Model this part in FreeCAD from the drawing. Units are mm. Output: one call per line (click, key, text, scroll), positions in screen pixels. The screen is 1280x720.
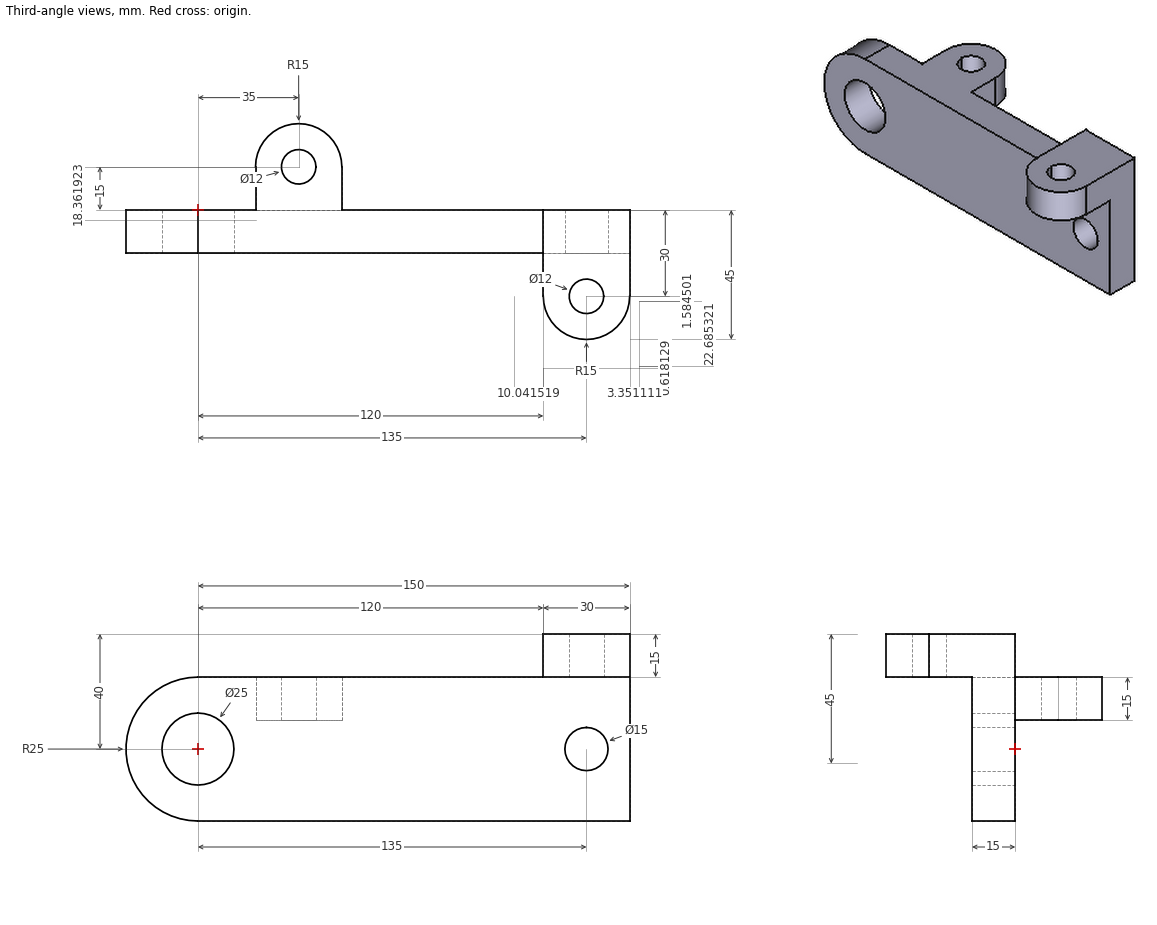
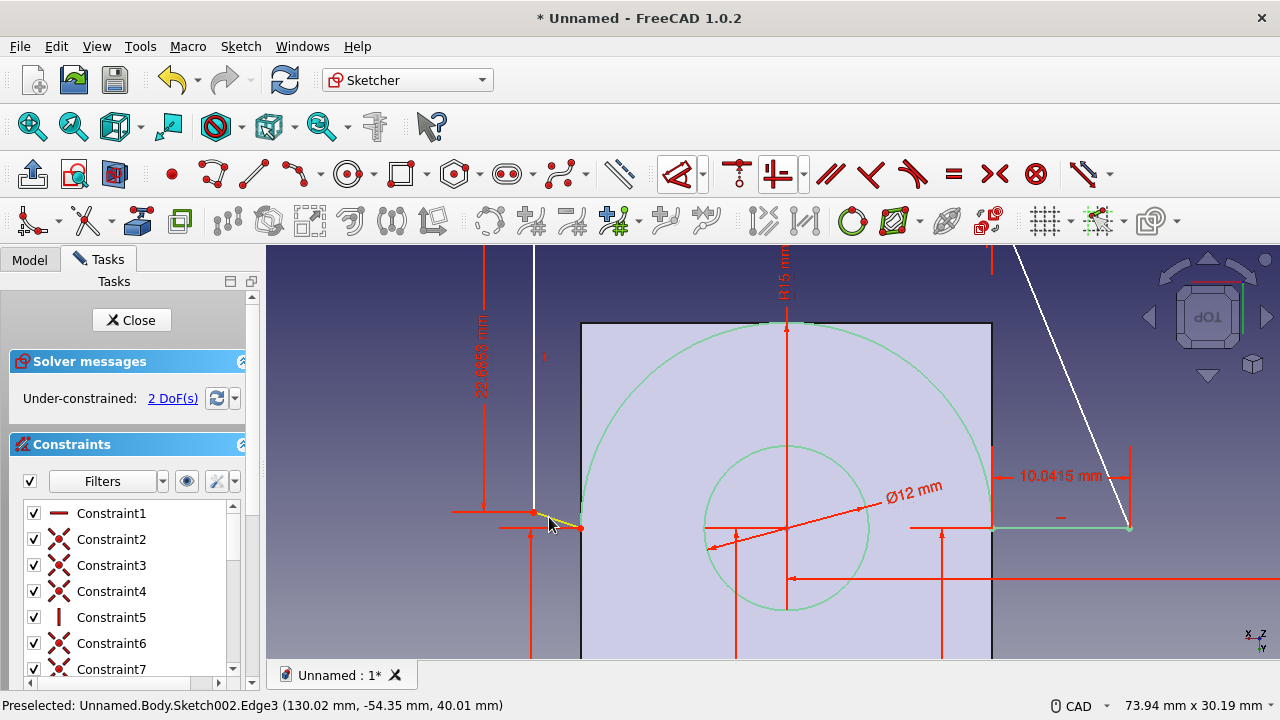
click(548, 517)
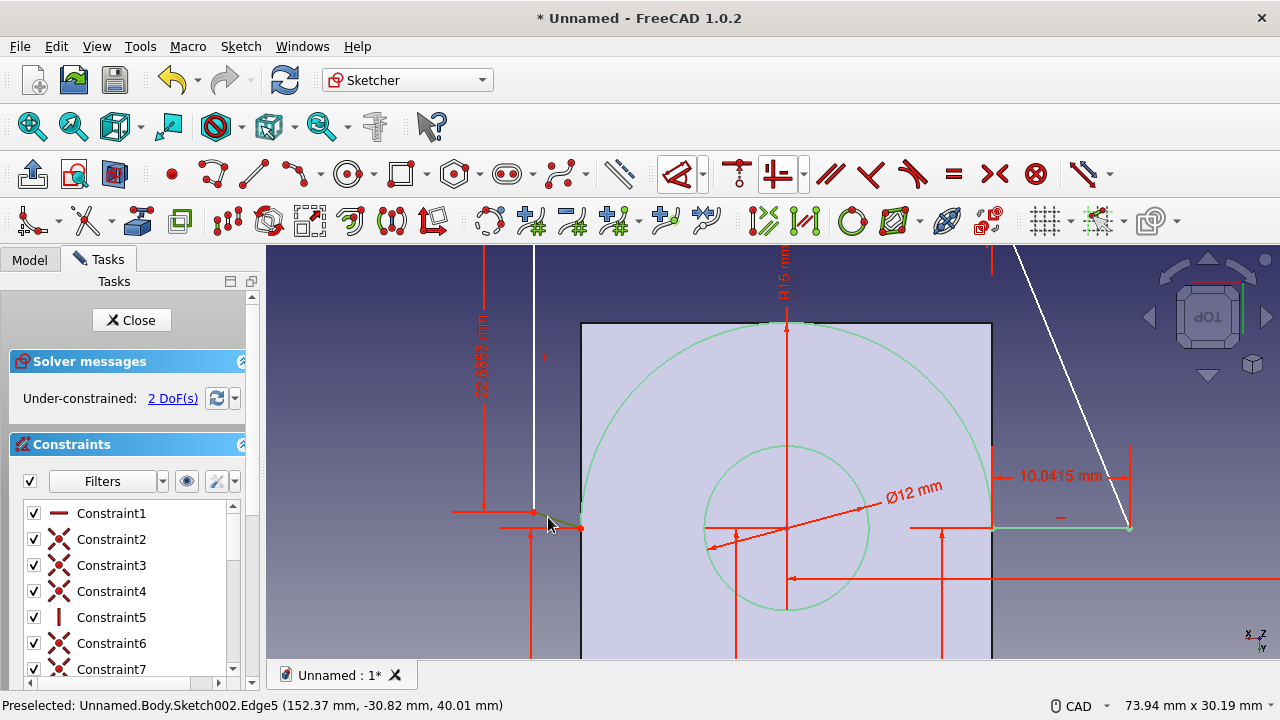
click(702, 174)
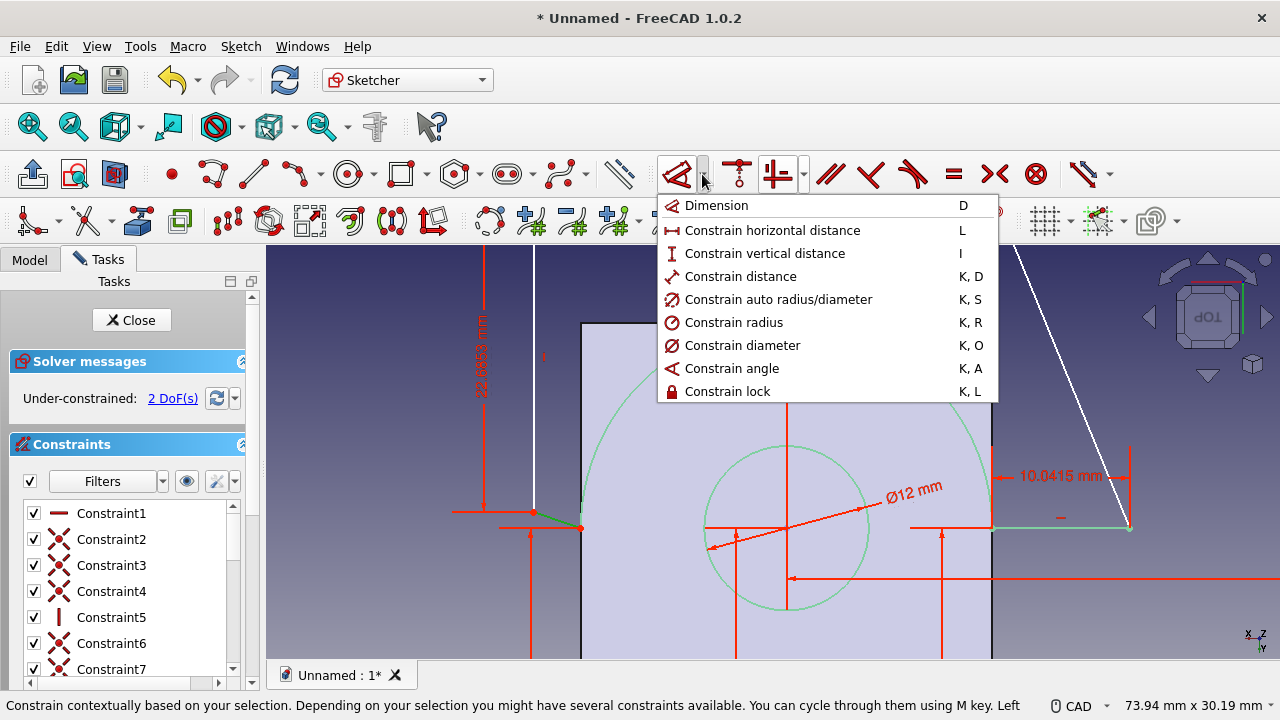
click(828, 230)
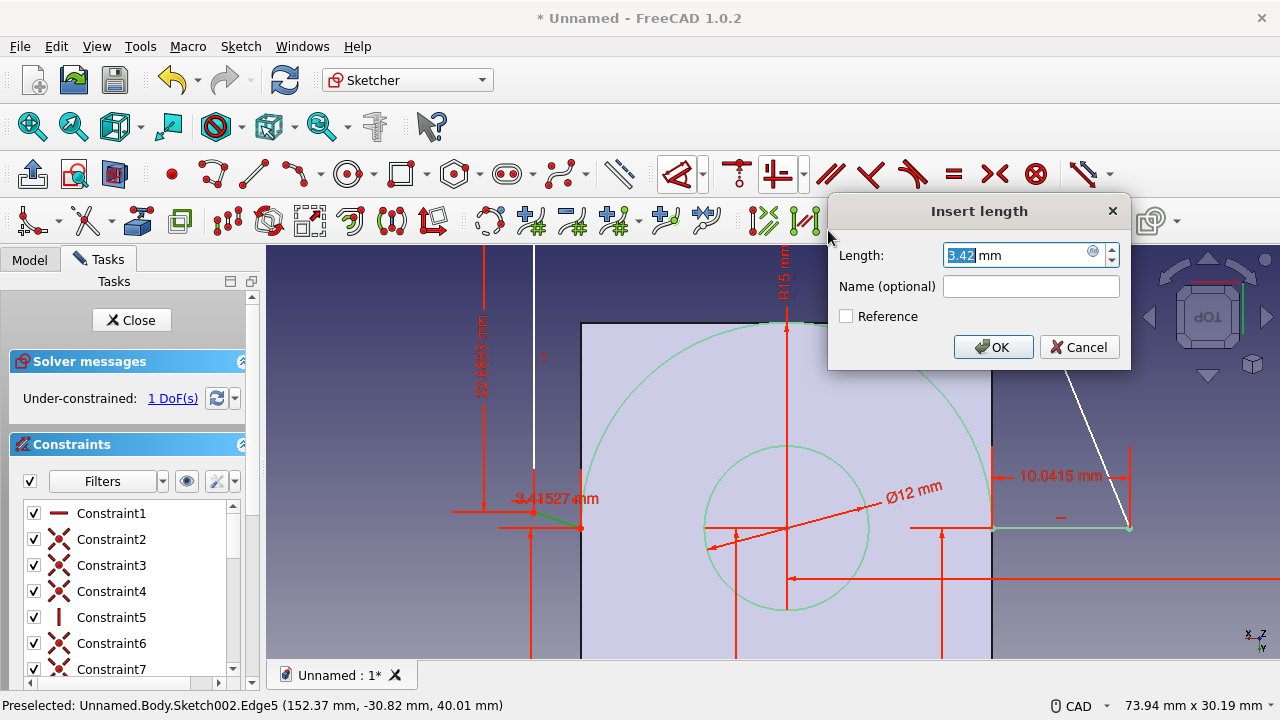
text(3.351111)
key(Return)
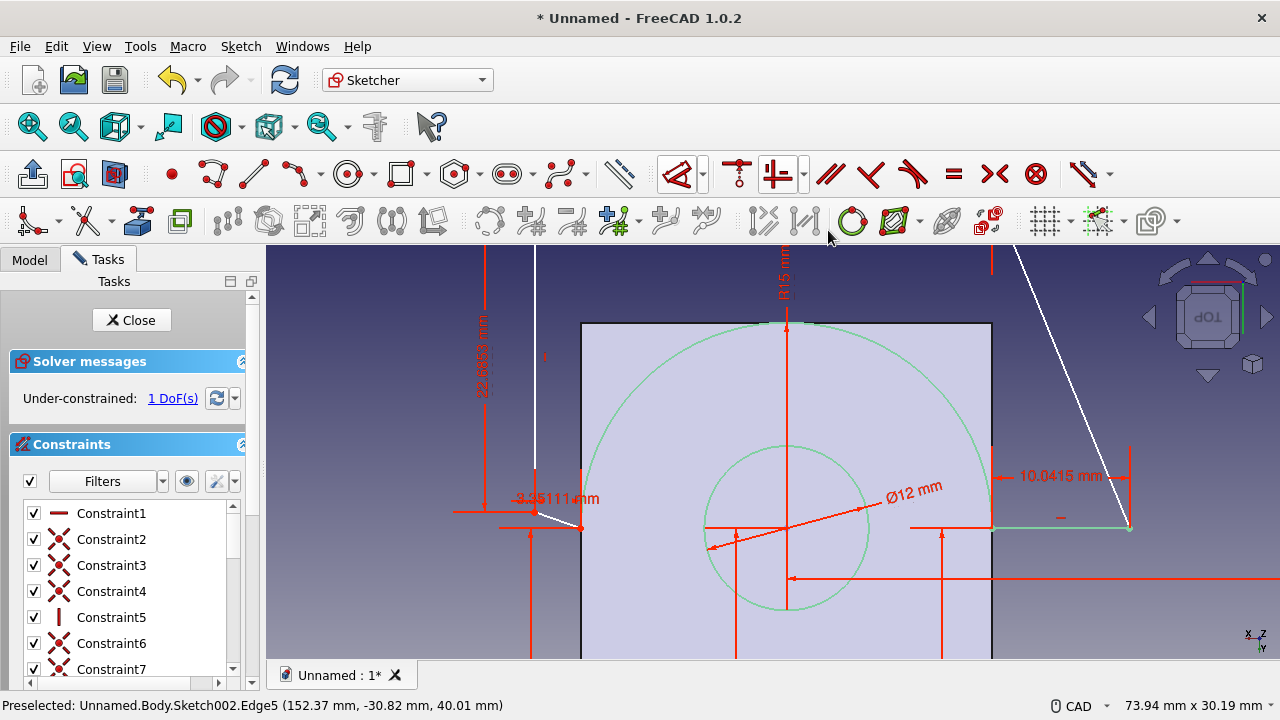
scroll(549, 517, up, 4)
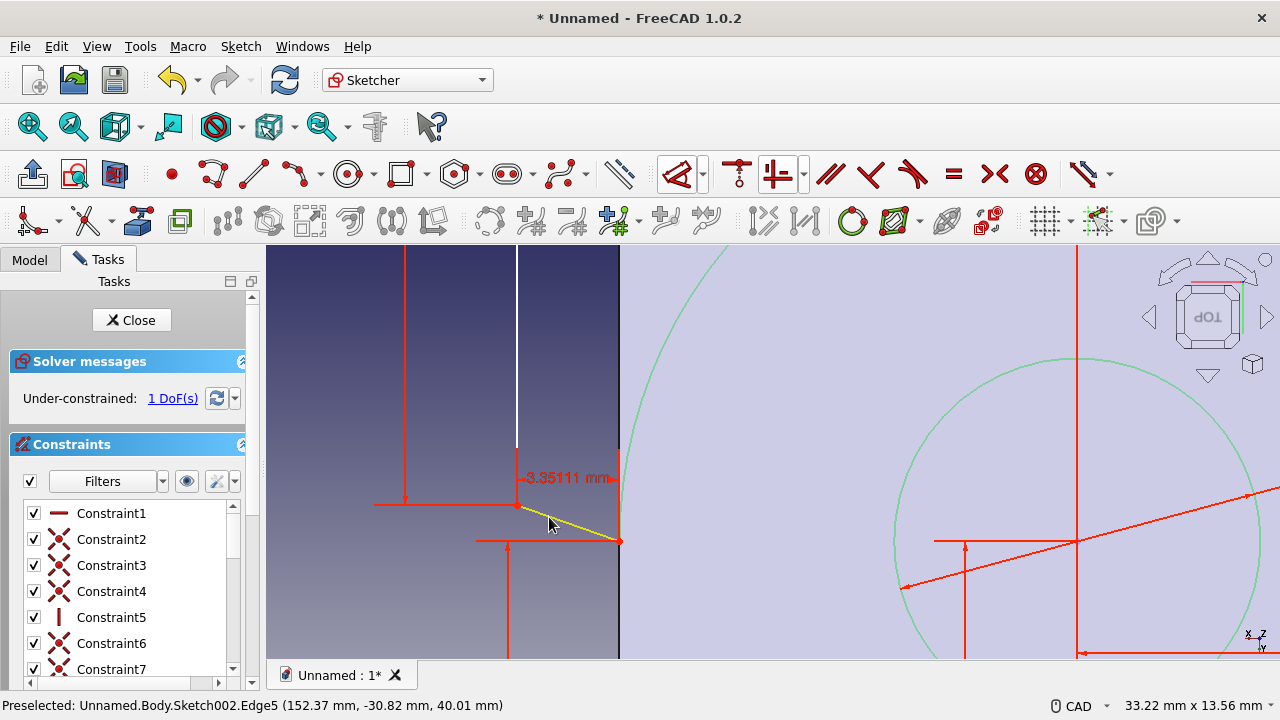
click(548, 516)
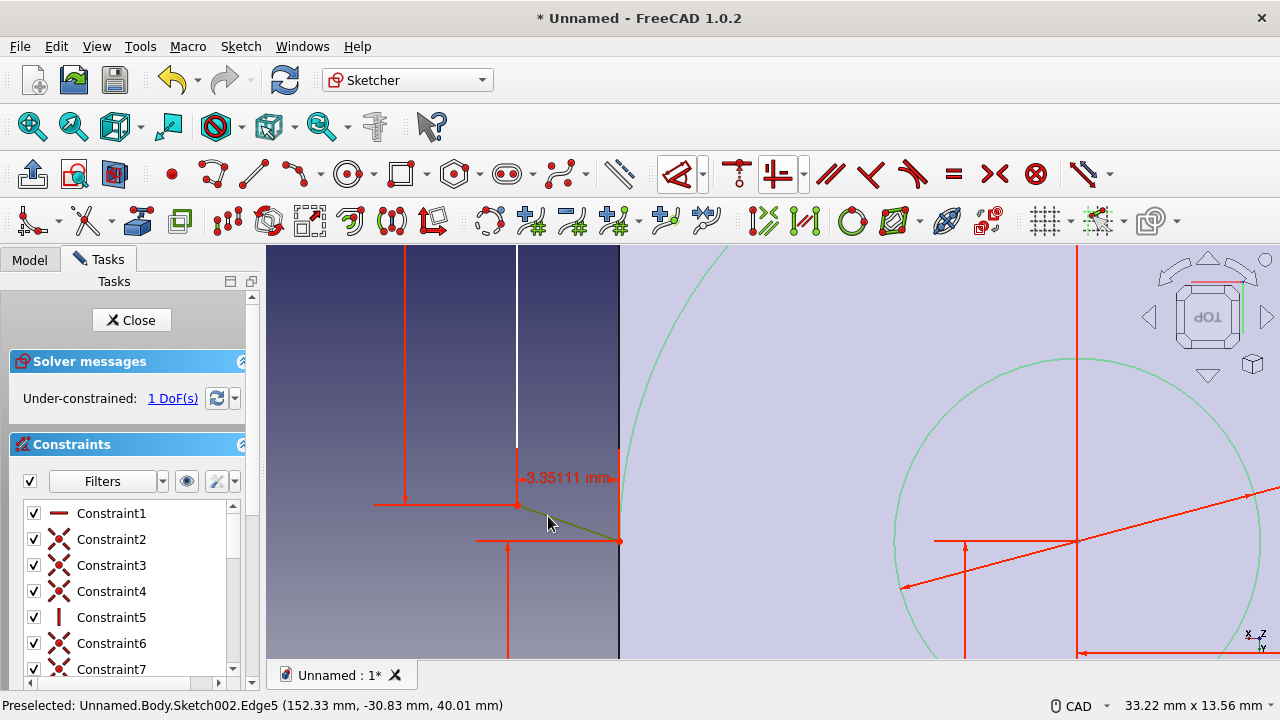
click(702, 174)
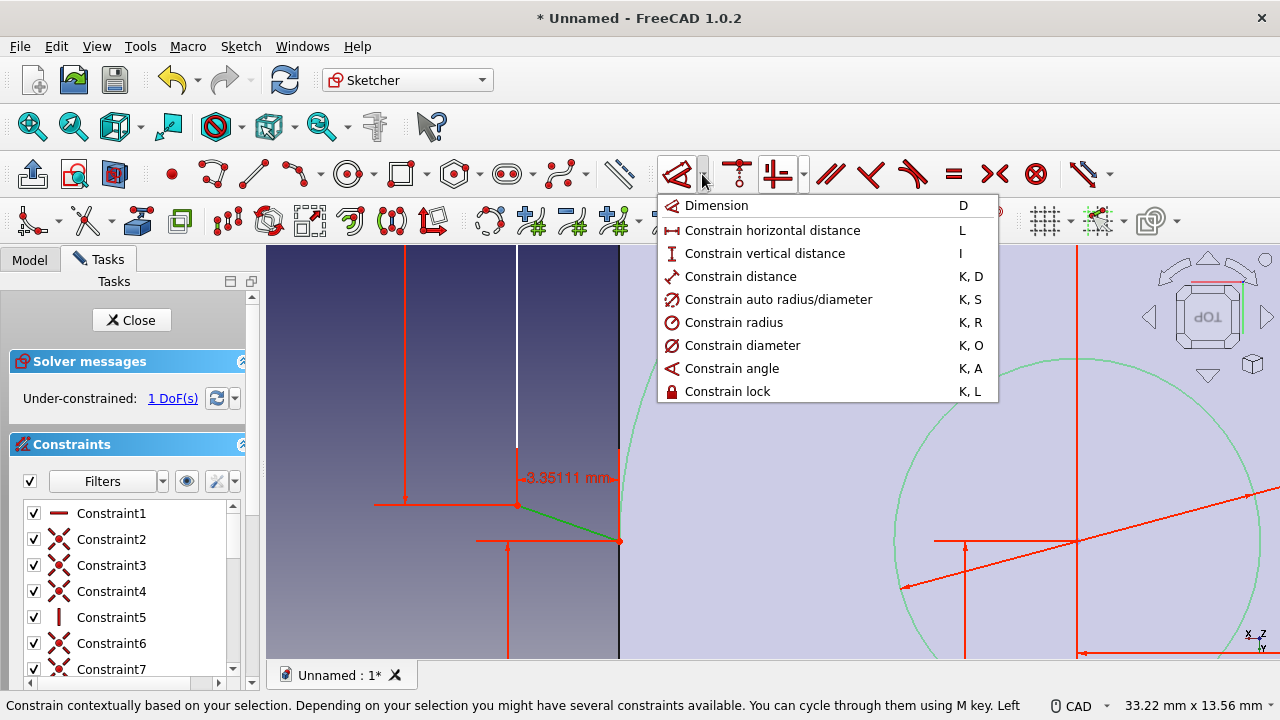
click(828, 254)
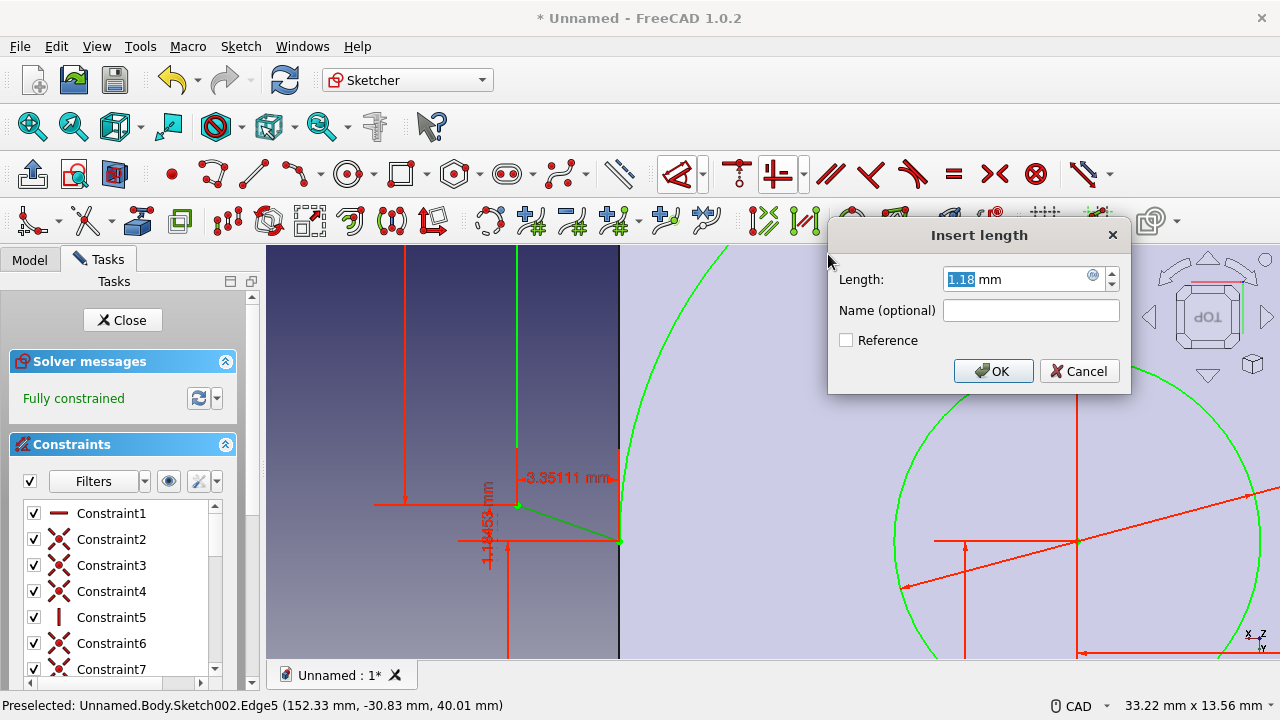
text(1.584501)
key(Return)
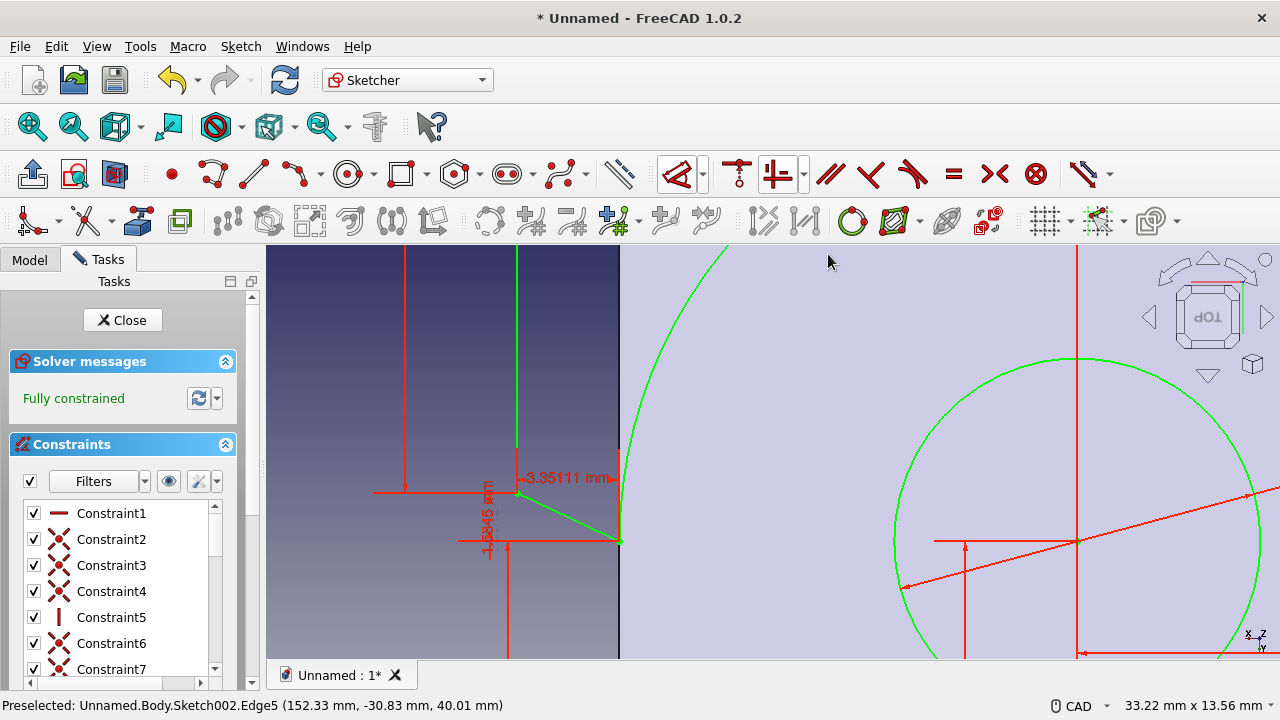
click(123, 320)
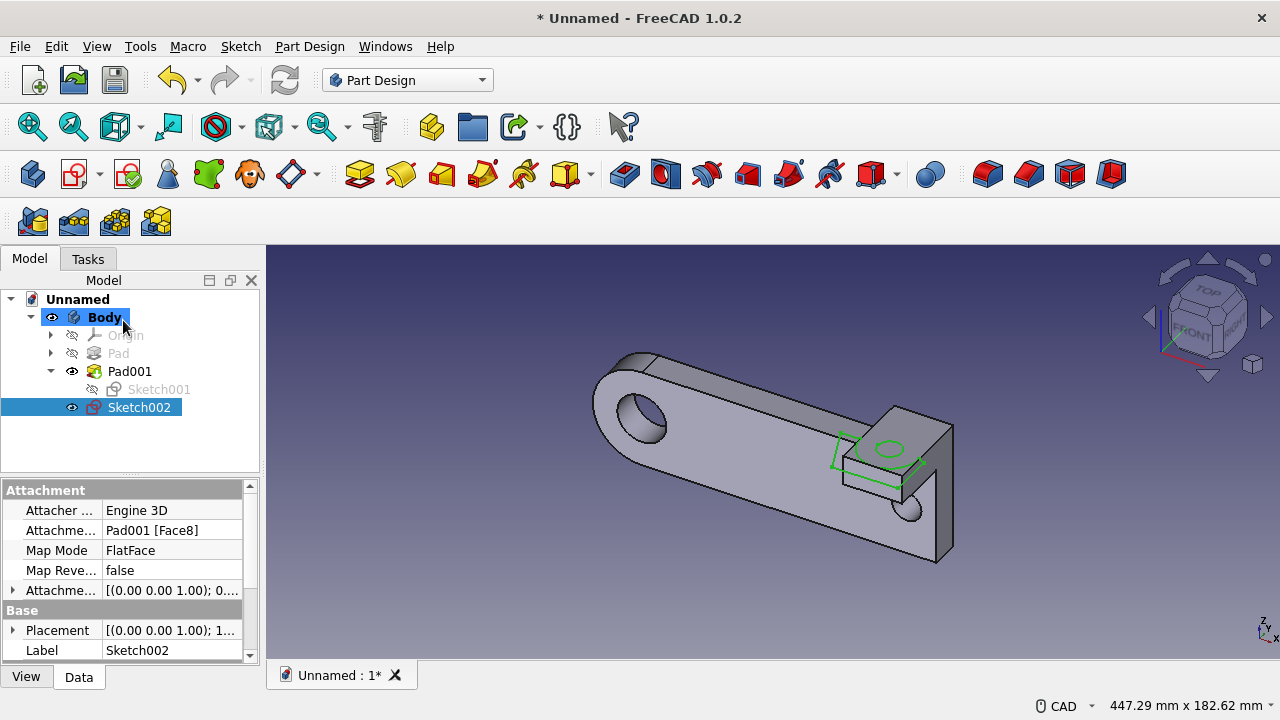
click(625, 174)